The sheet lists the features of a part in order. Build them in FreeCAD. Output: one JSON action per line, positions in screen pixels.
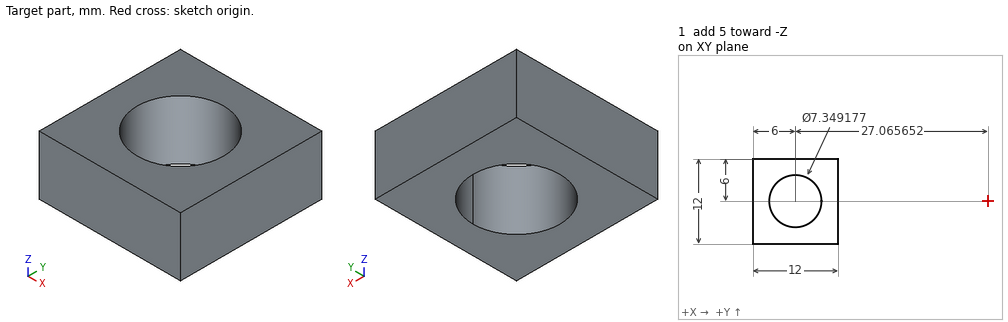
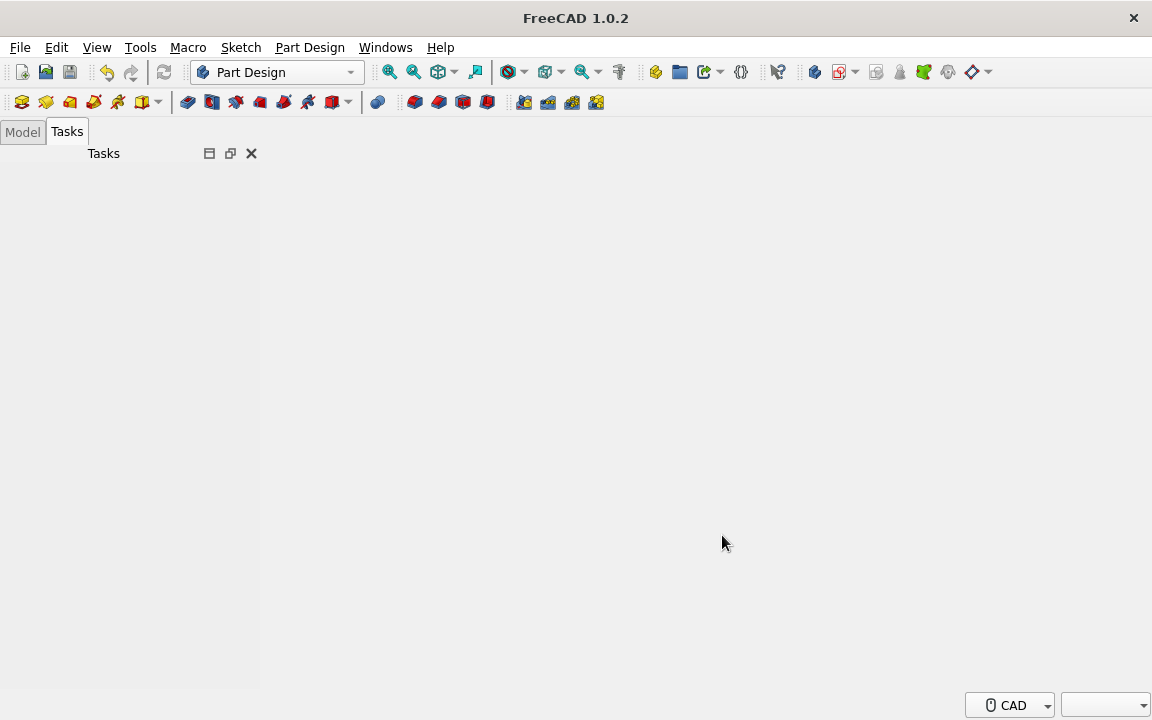
{"action": "left_click", "coordinate": [22, 72]}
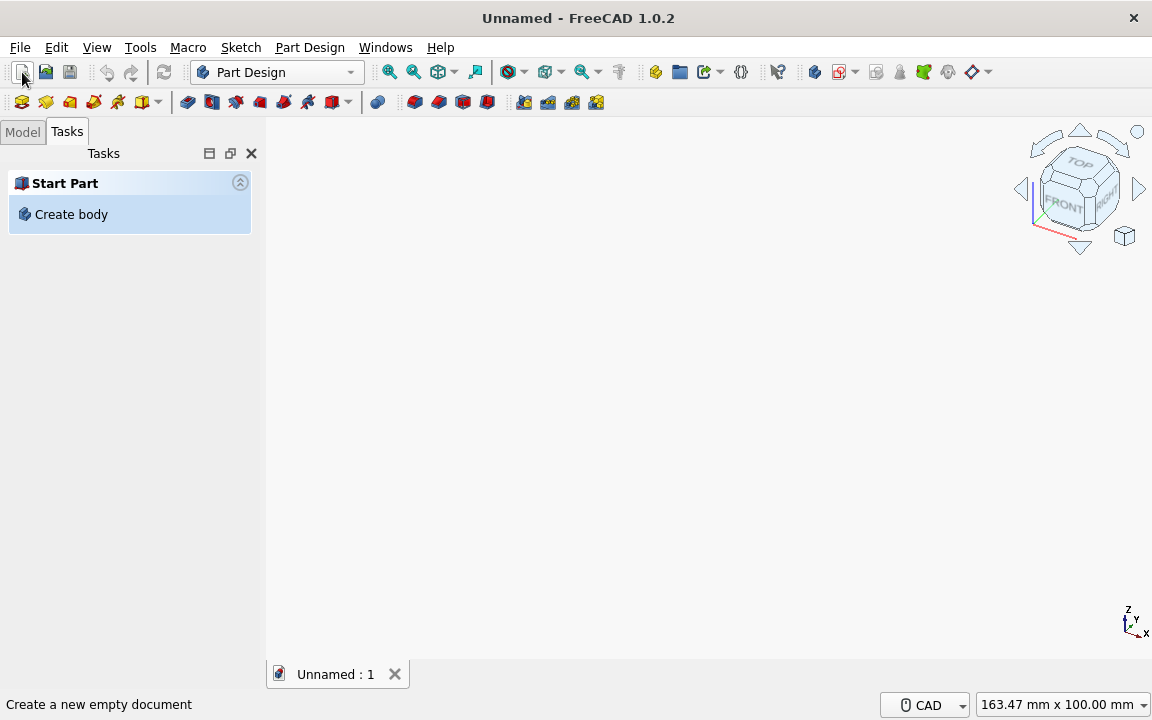
{"action": "left_click", "coordinate": [840, 72]}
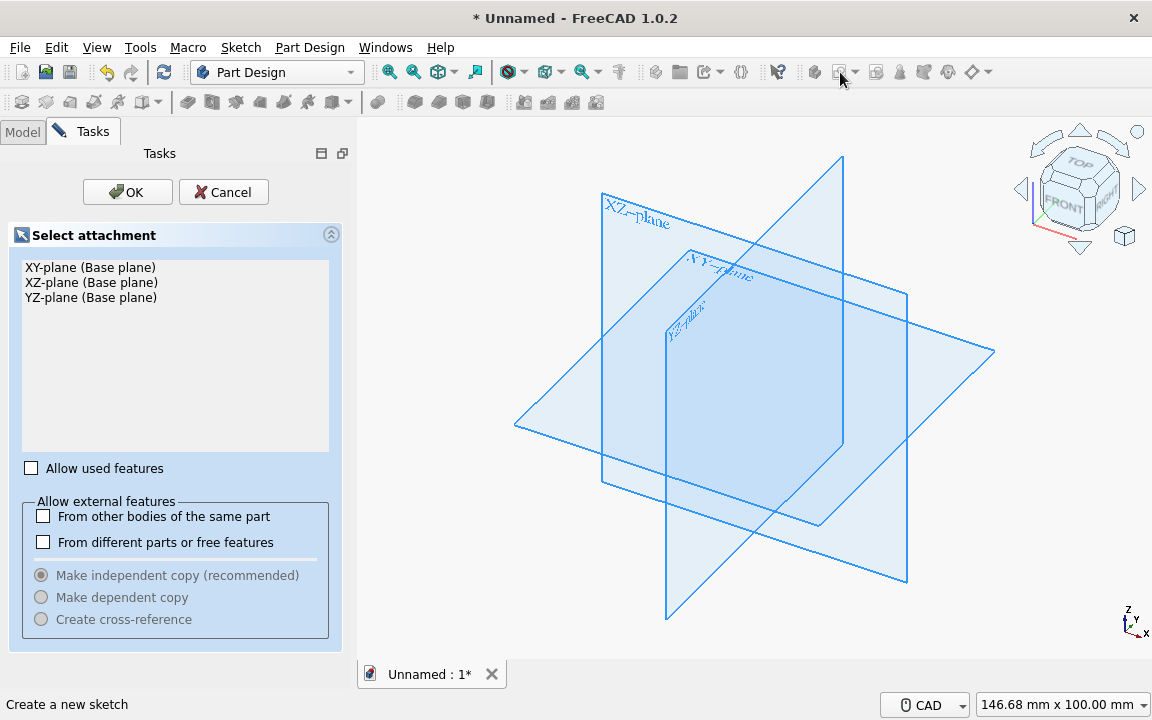
{"action": "left_click", "coordinate": [82, 268]}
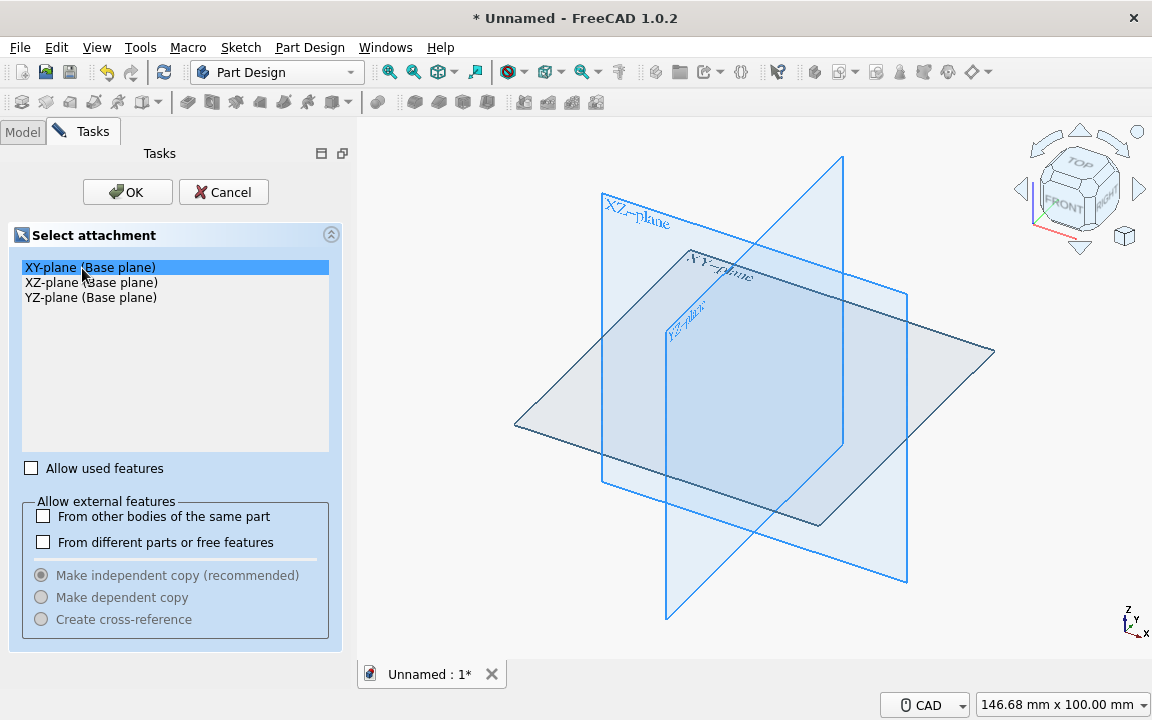
{"action": "left_click", "coordinate": [128, 192]}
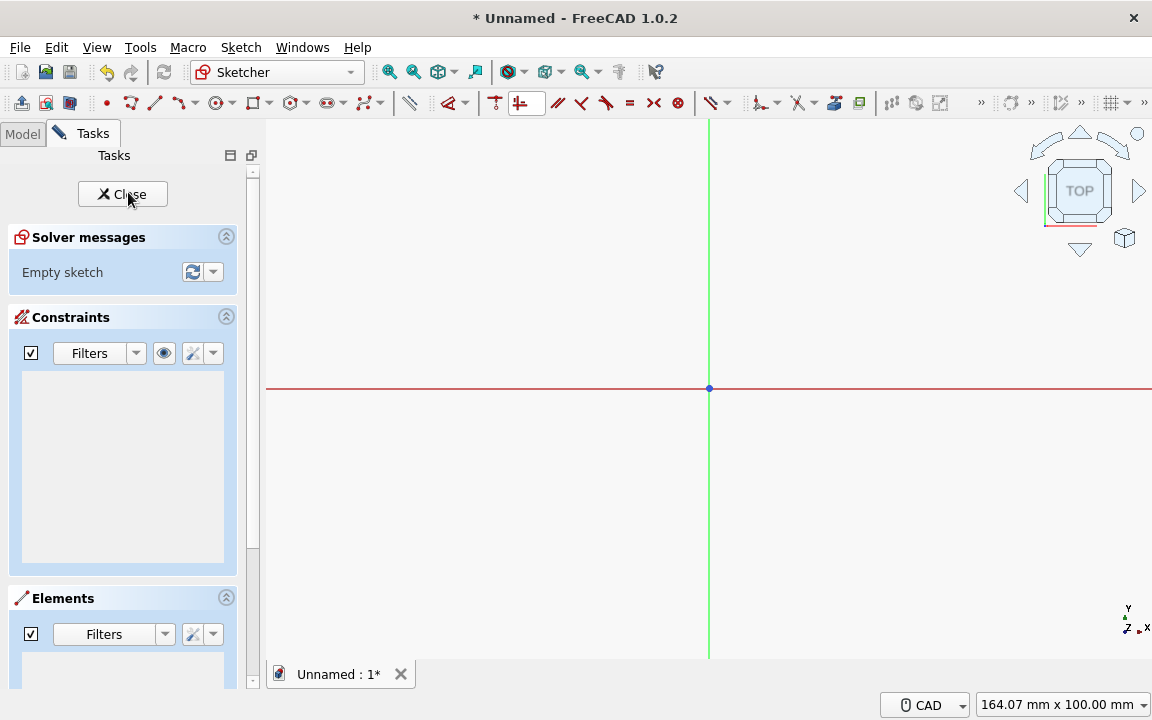
{"action": "scroll", "coordinate": [543, 389], "scroll_direction": "up", "scroll_amount": 8}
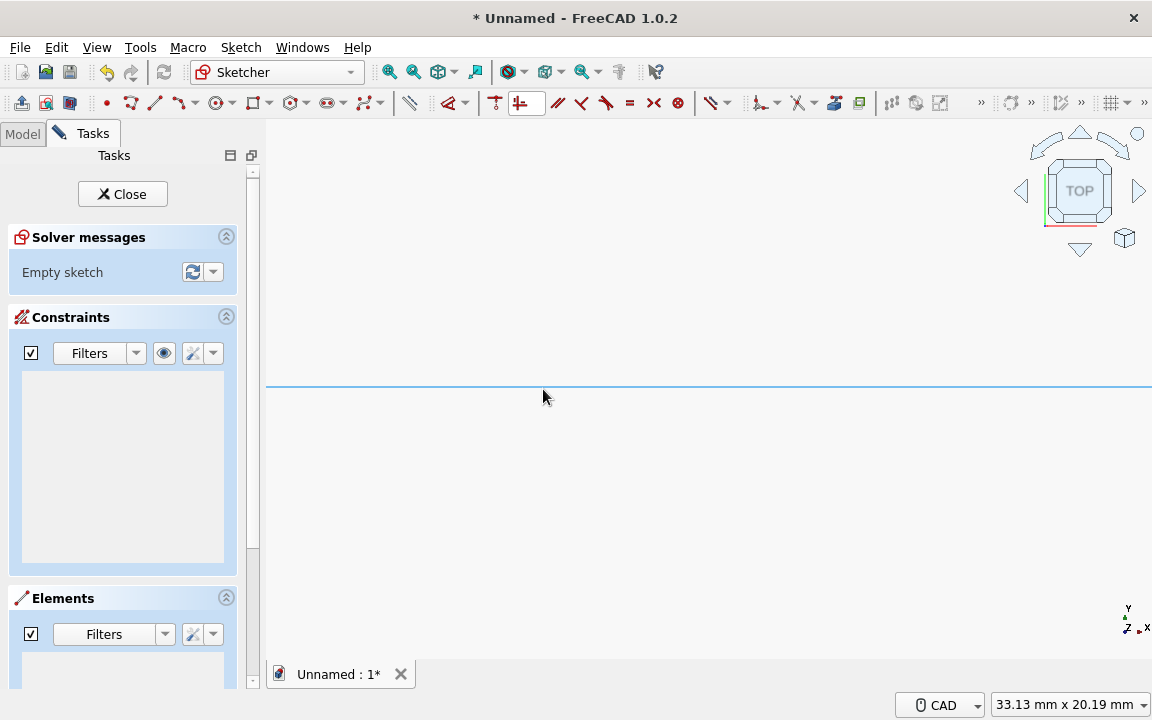
{"action": "key", "text": "g r"}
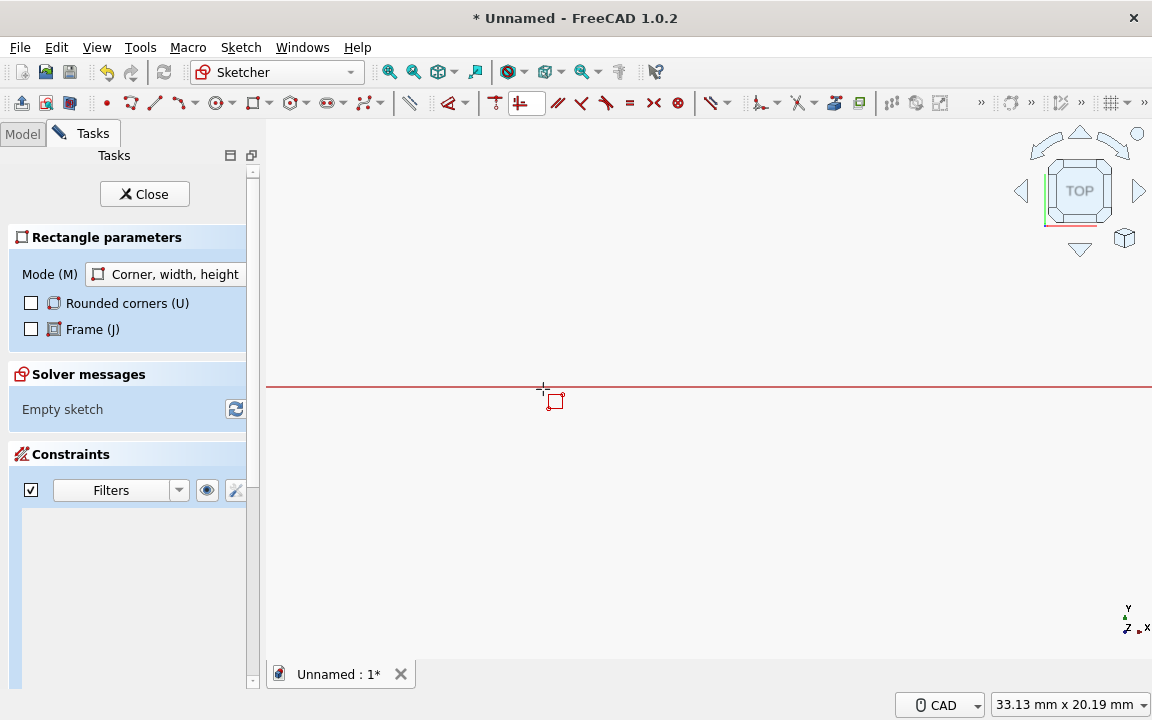
{"action": "left_click", "coordinate": [480, 227]}
{"action": "left_click", "coordinate": [801, 547]}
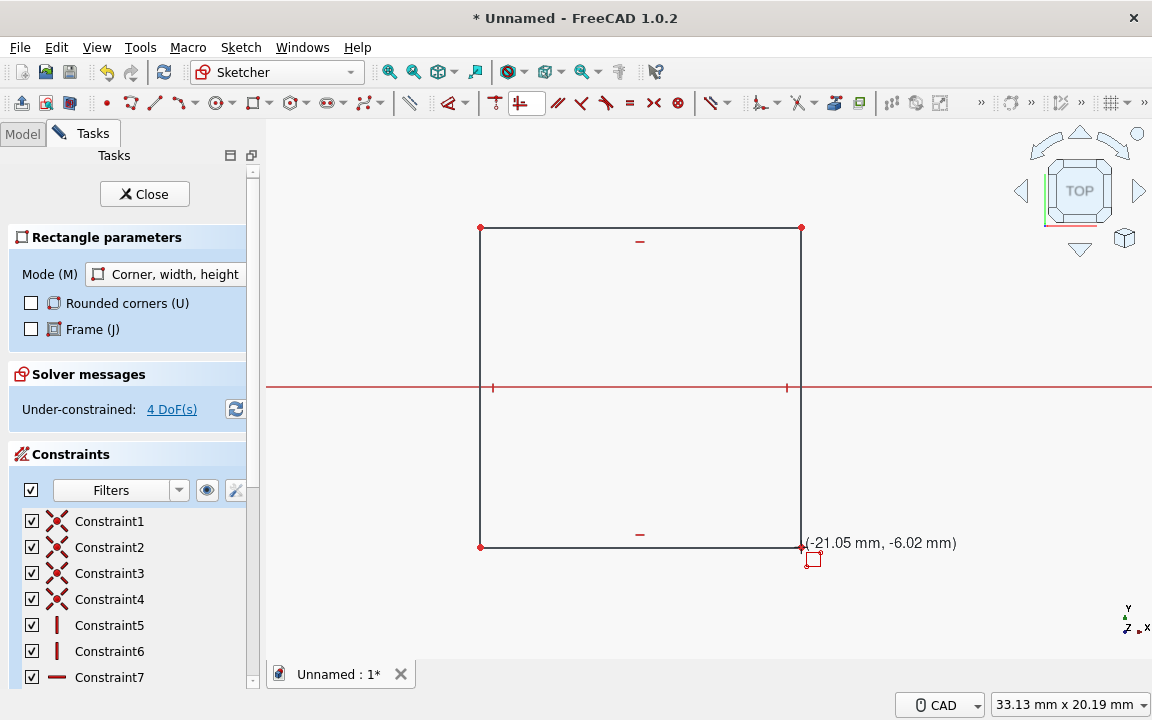
{"action": "key", "text": "g c"}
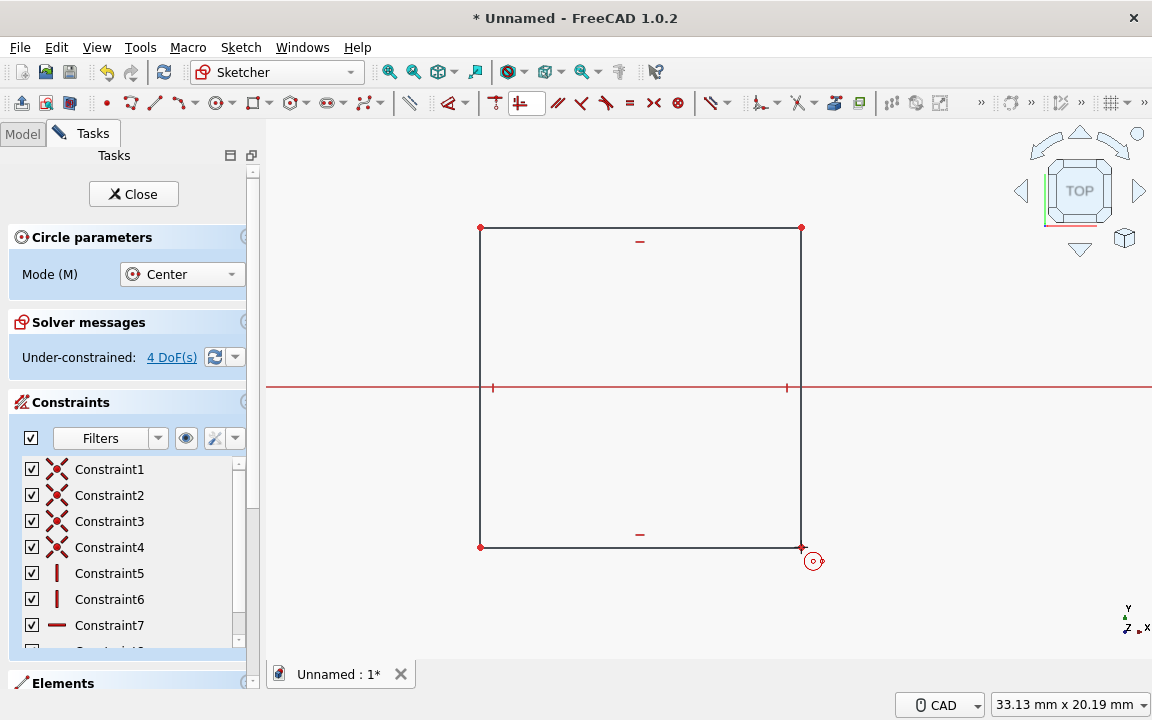
{"action": "left_click", "coordinate": [640, 387]}
{"action": "left_click", "coordinate": [710, 318]}
{"action": "key", "text": "Escape"}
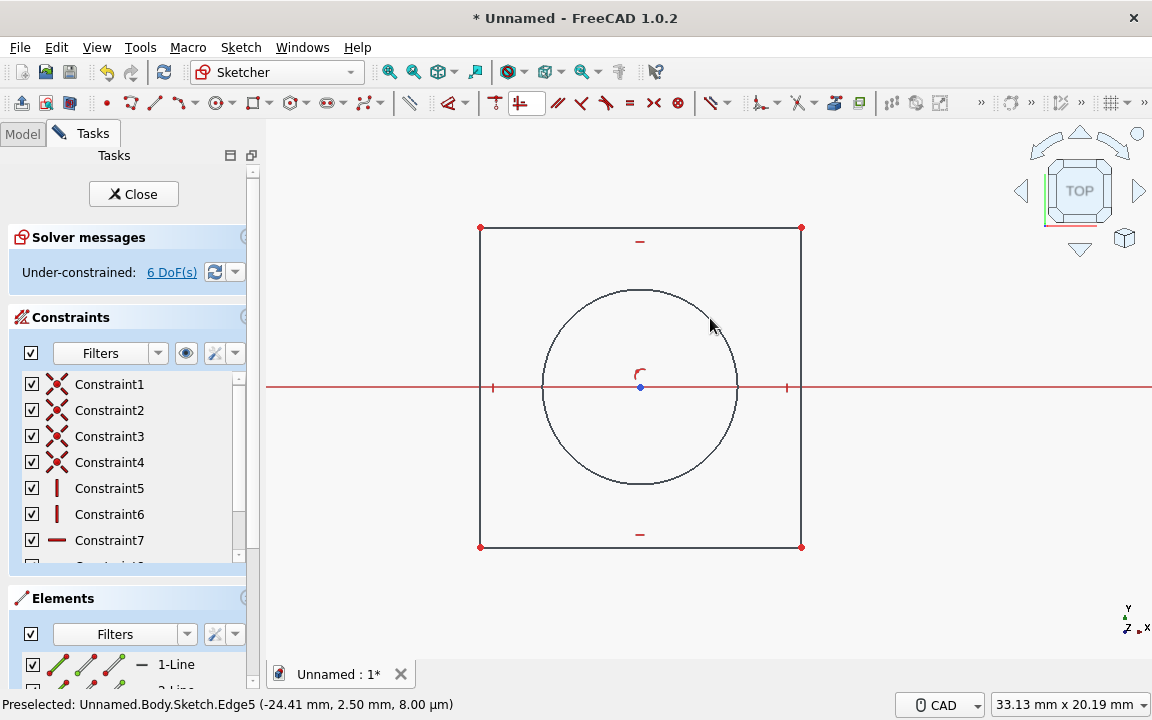
{"action": "key", "text": "d"}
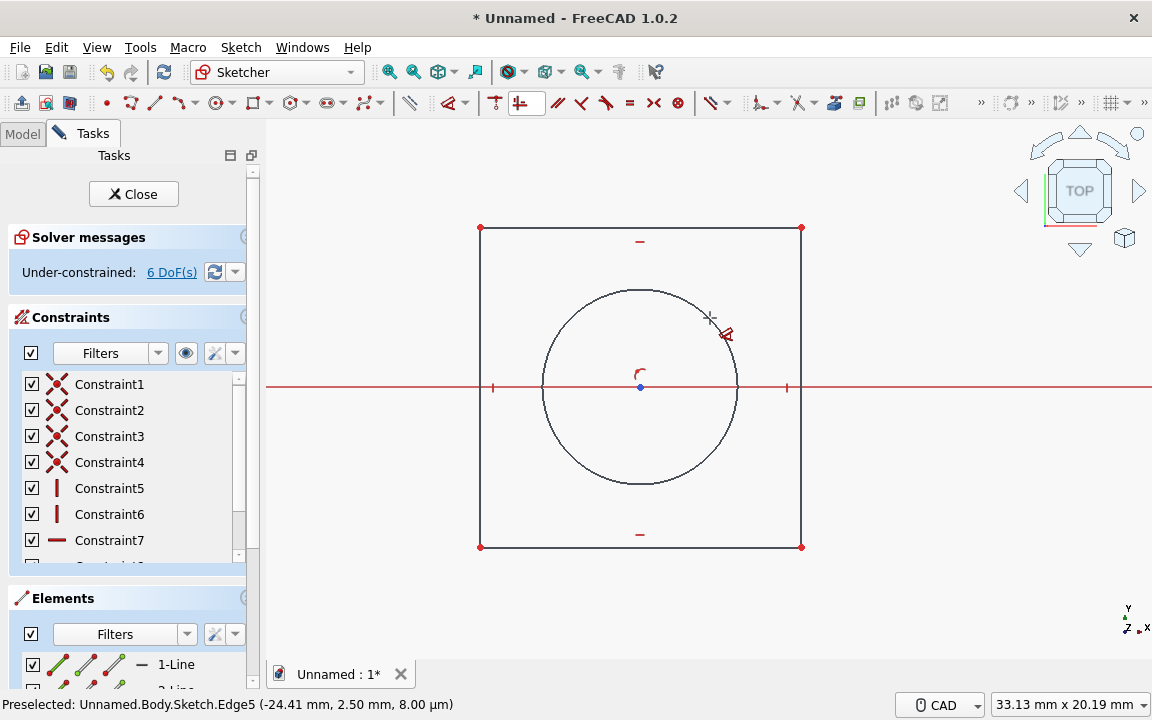
{"action": "left_click", "coordinate": [709, 318]}
{"action": "left_click", "coordinate": [732, 295]}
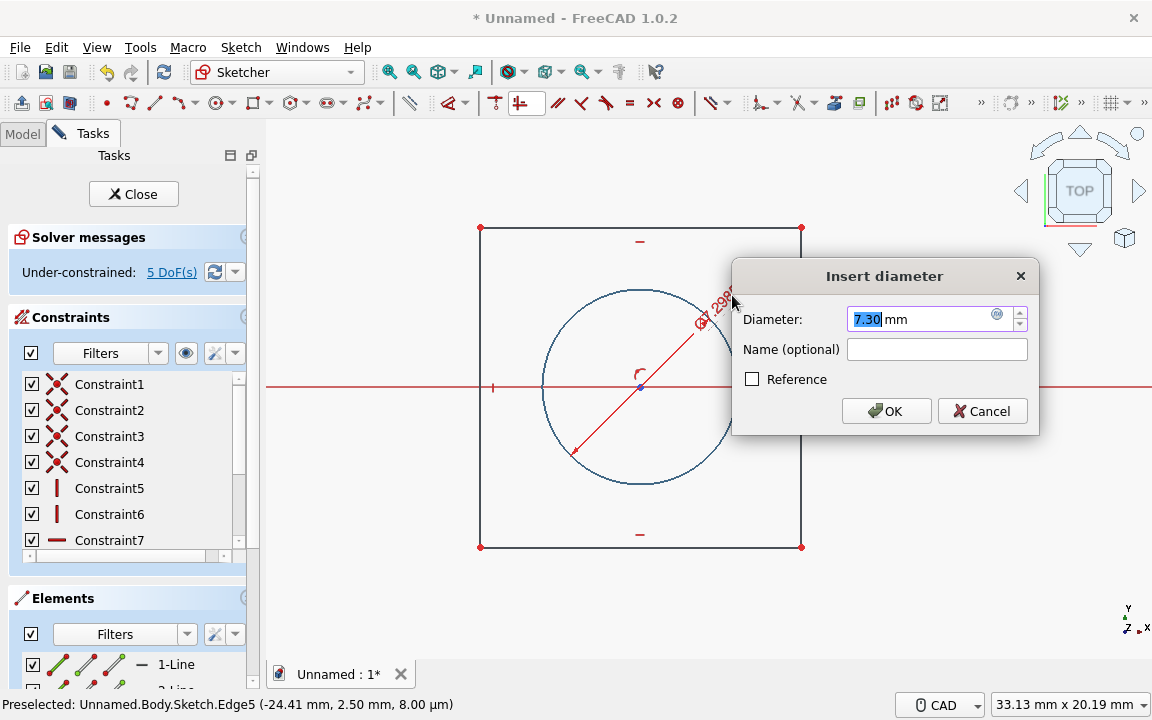
{"action": "type", "text": "7.349177"}
{"action": "key", "text": "Return"}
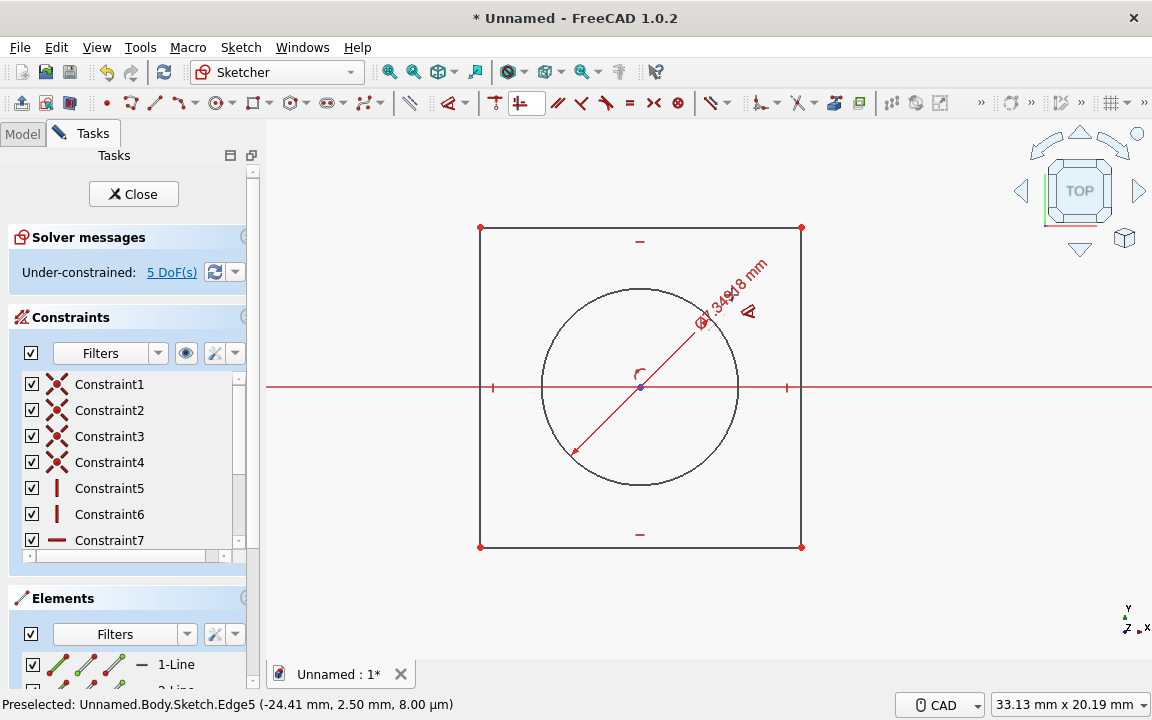
{"action": "left_click", "coordinate": [480, 324]}
{"action": "left_click", "coordinate": [446, 314]}